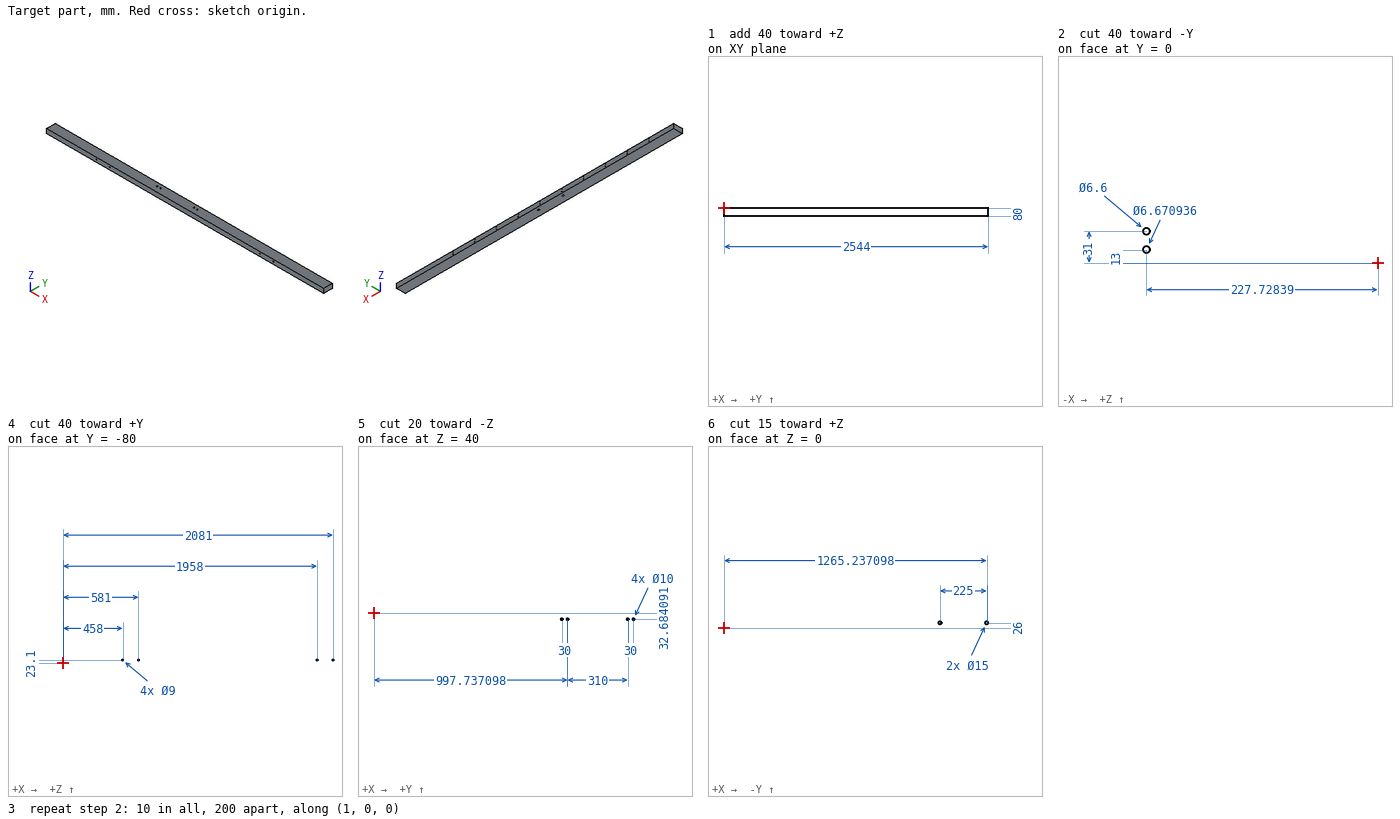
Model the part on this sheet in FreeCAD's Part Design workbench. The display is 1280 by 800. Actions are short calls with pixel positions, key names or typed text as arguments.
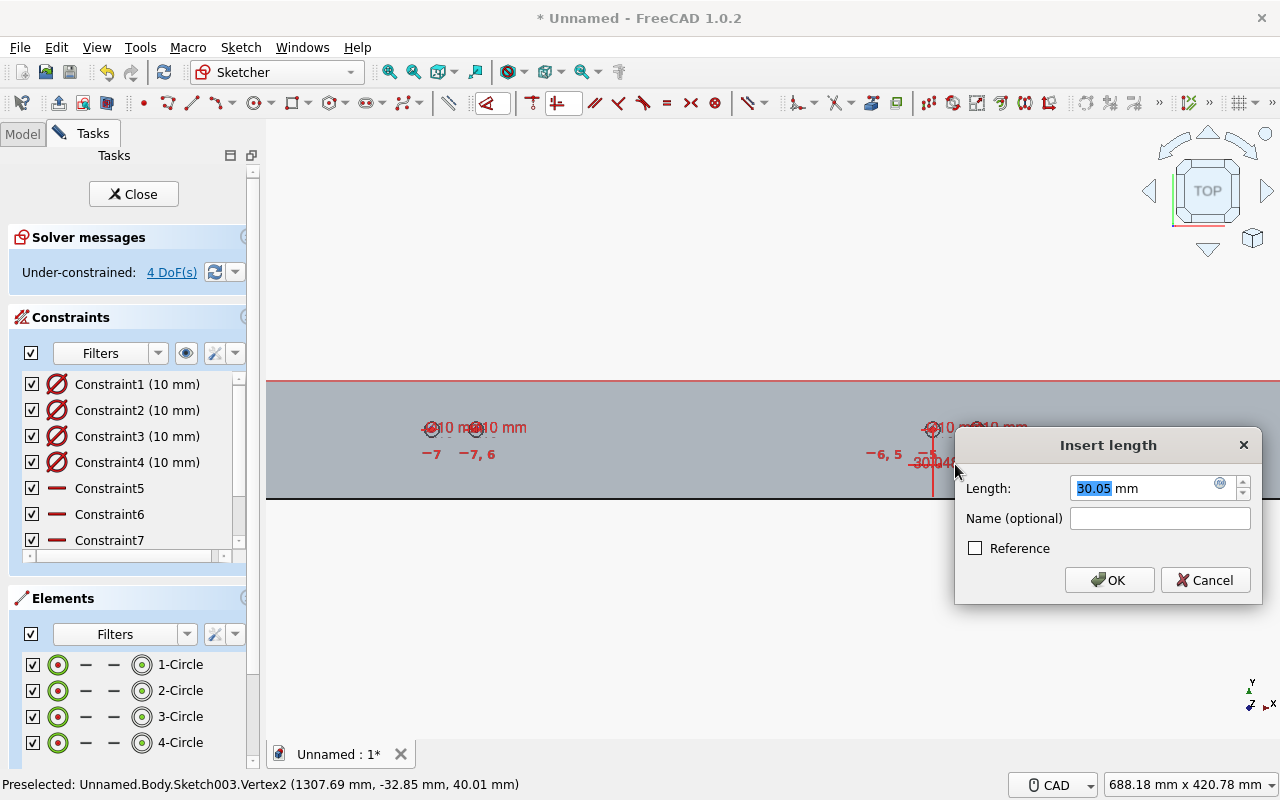
text(30)
key(Return)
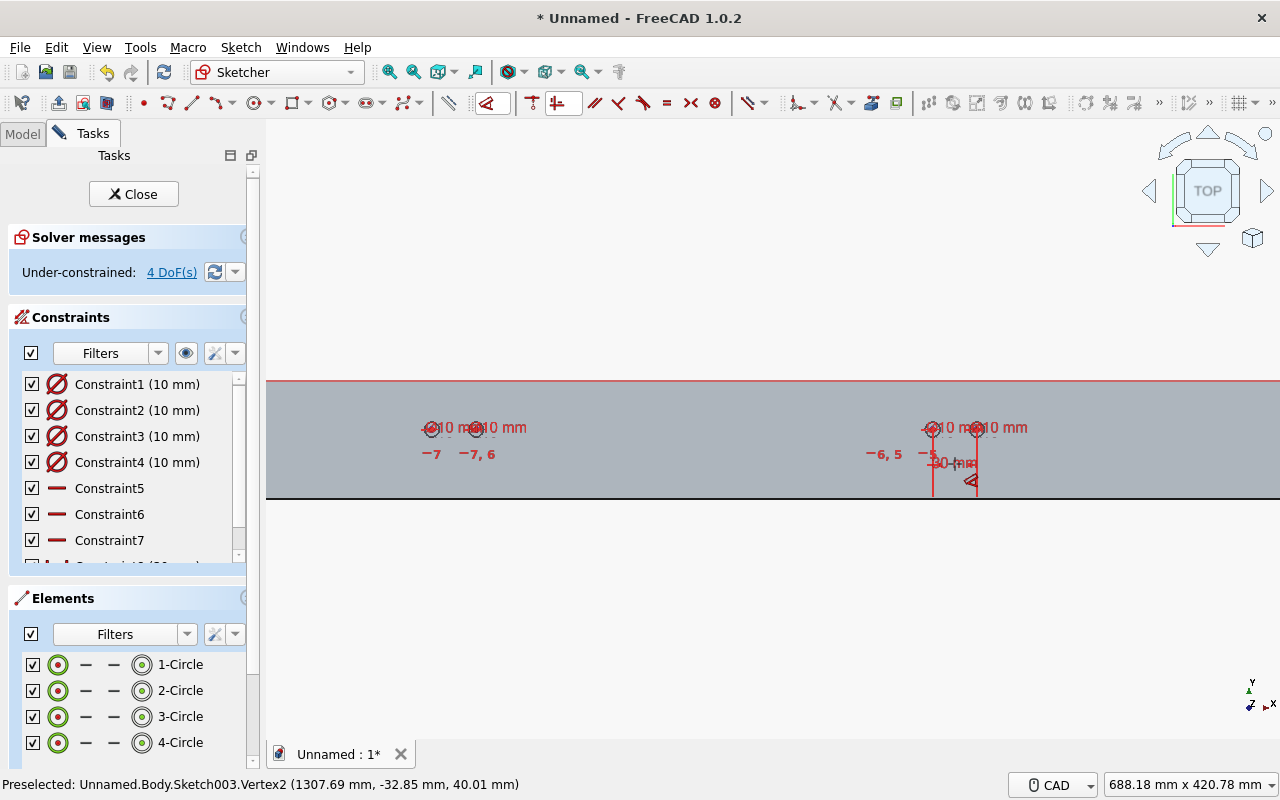
click(476, 430)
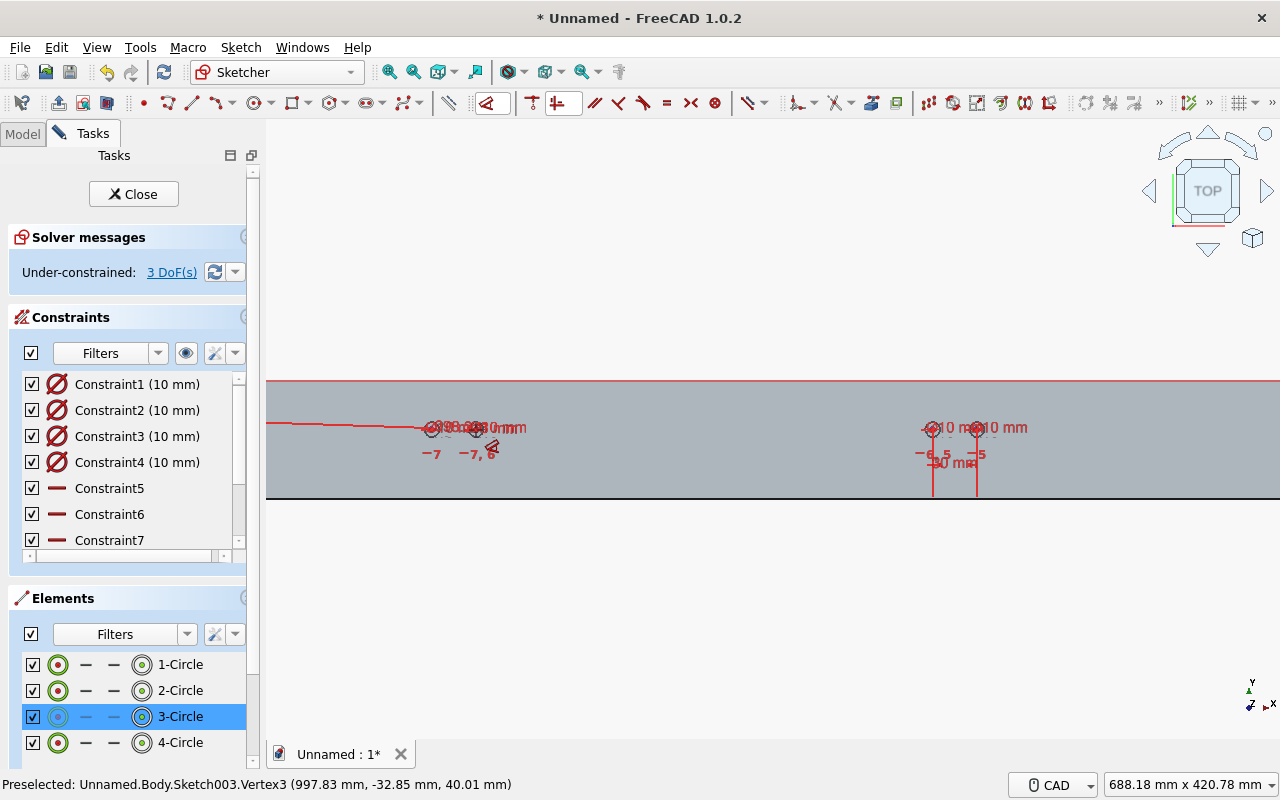
click(432, 430)
click(454, 464)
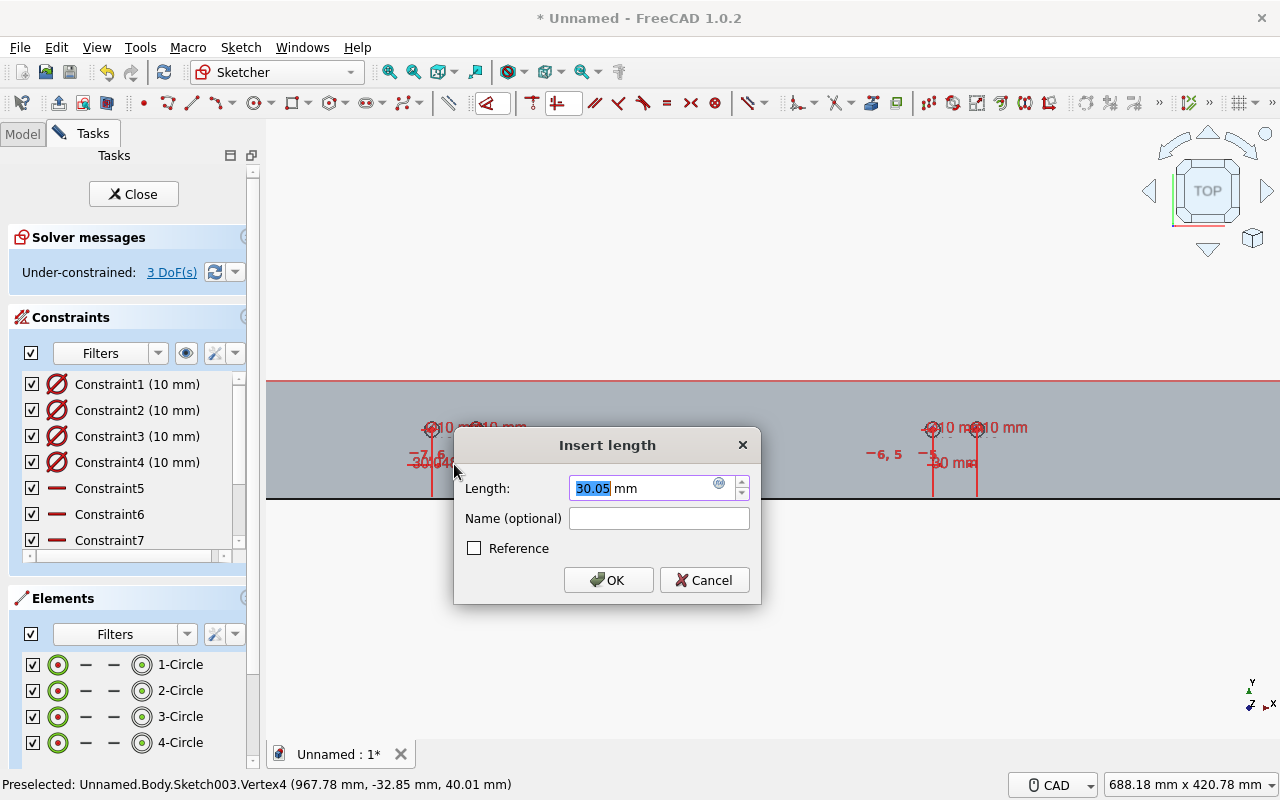
text(30)
key(Return)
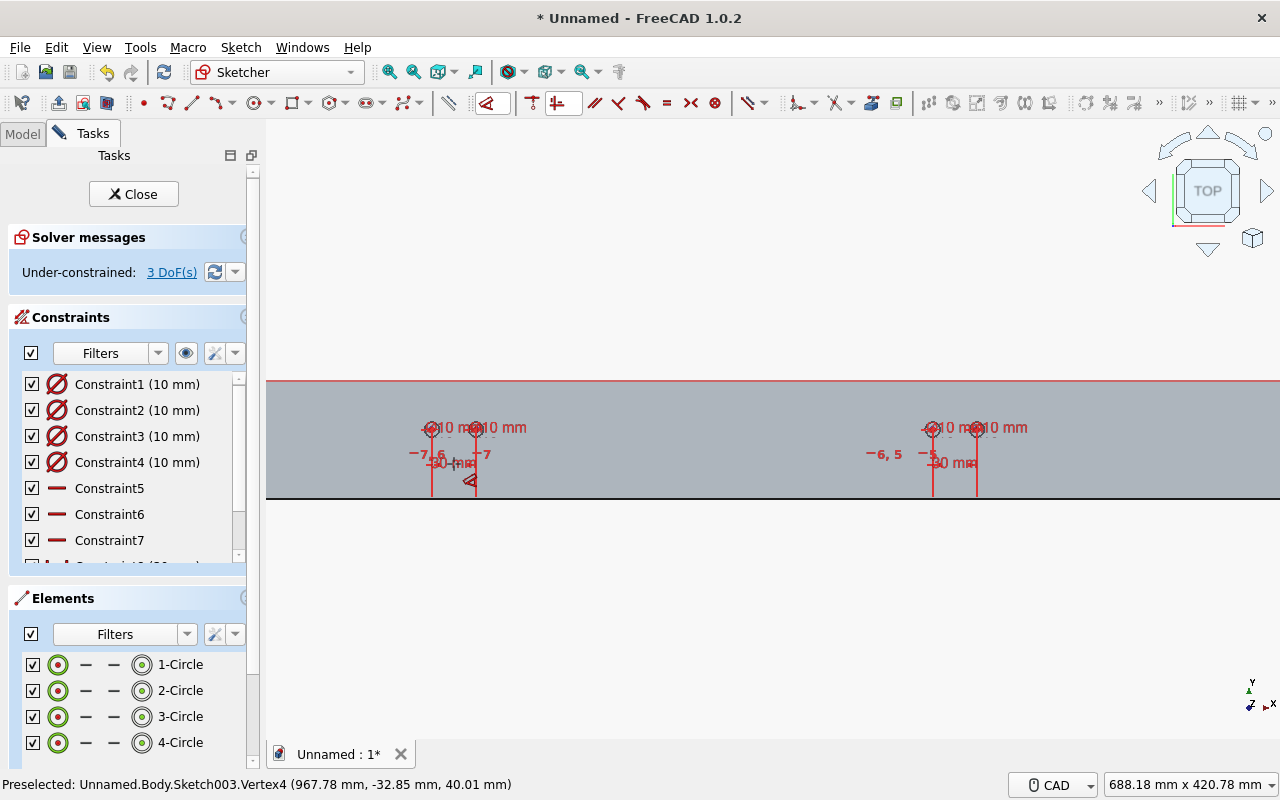
click(933, 430)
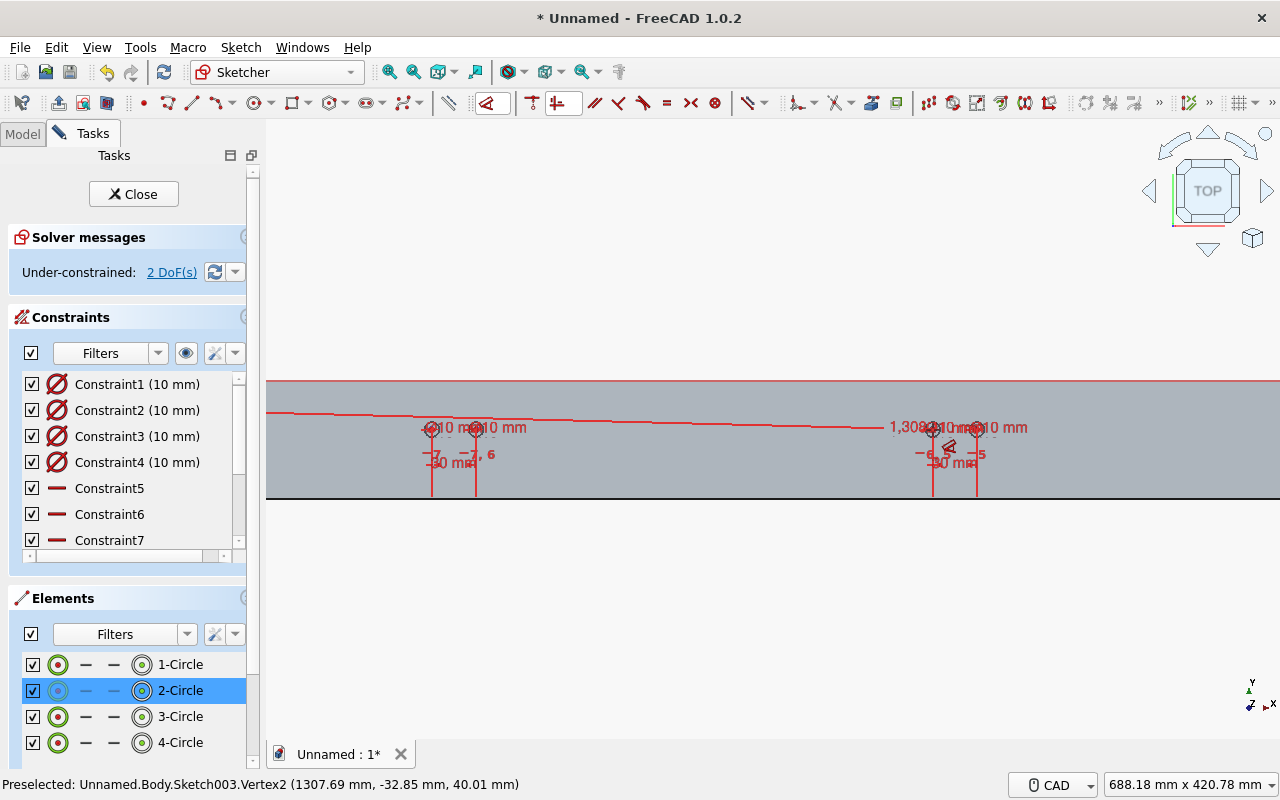
click(476, 430)
click(704, 464)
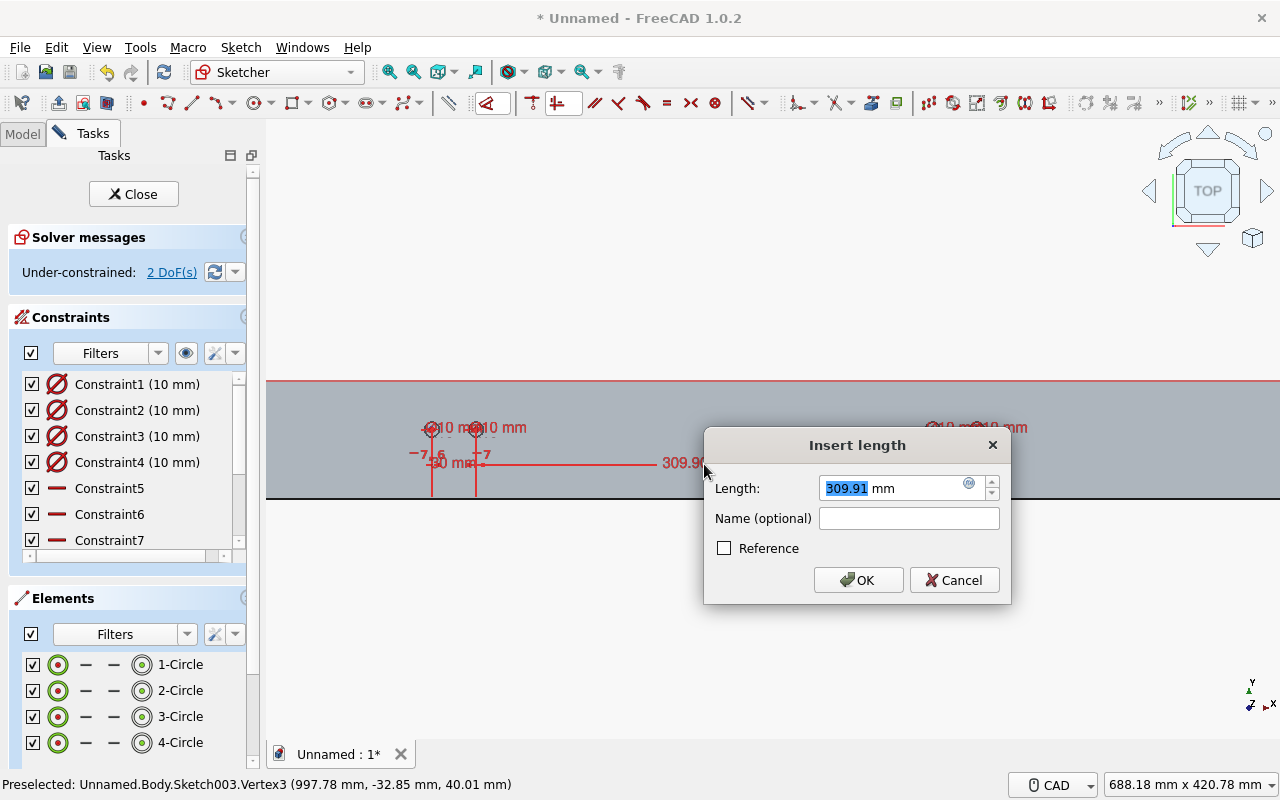
text(310)
key(Return)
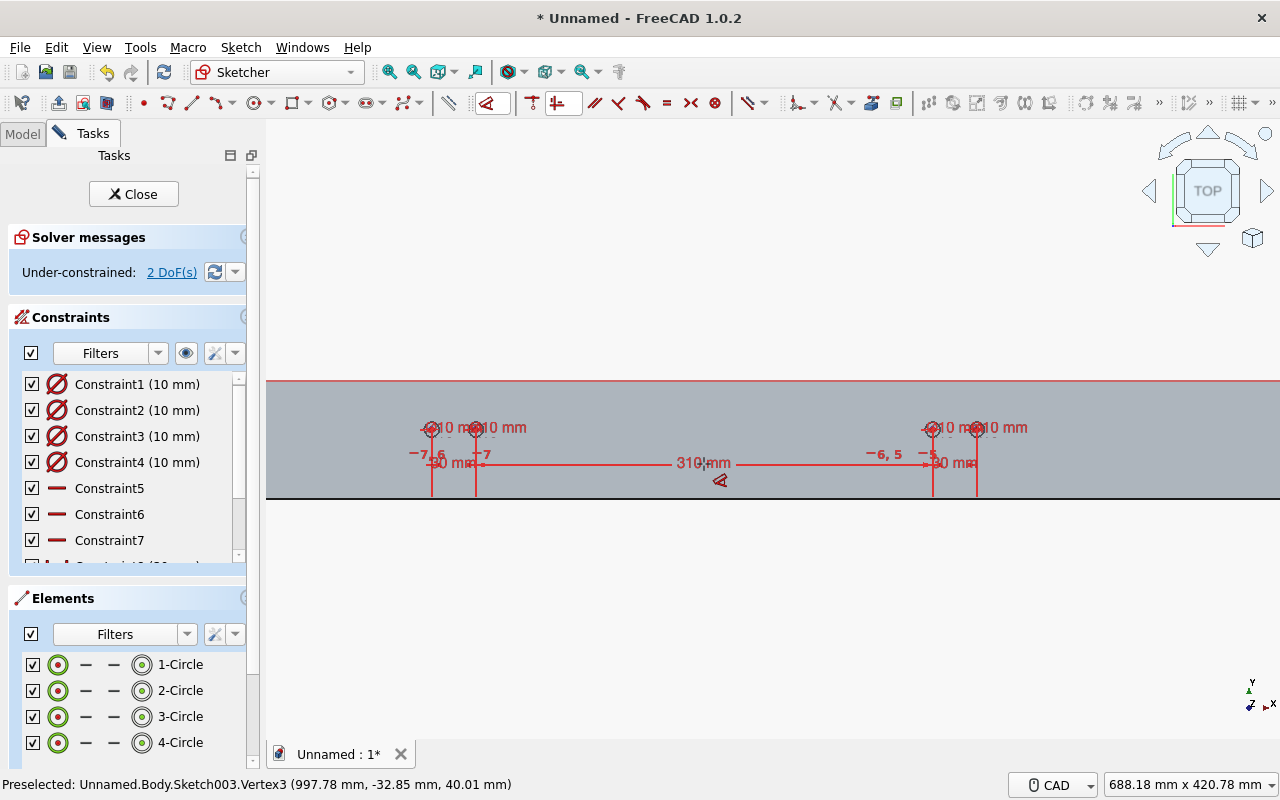
click(977, 430)
click(1011, 405)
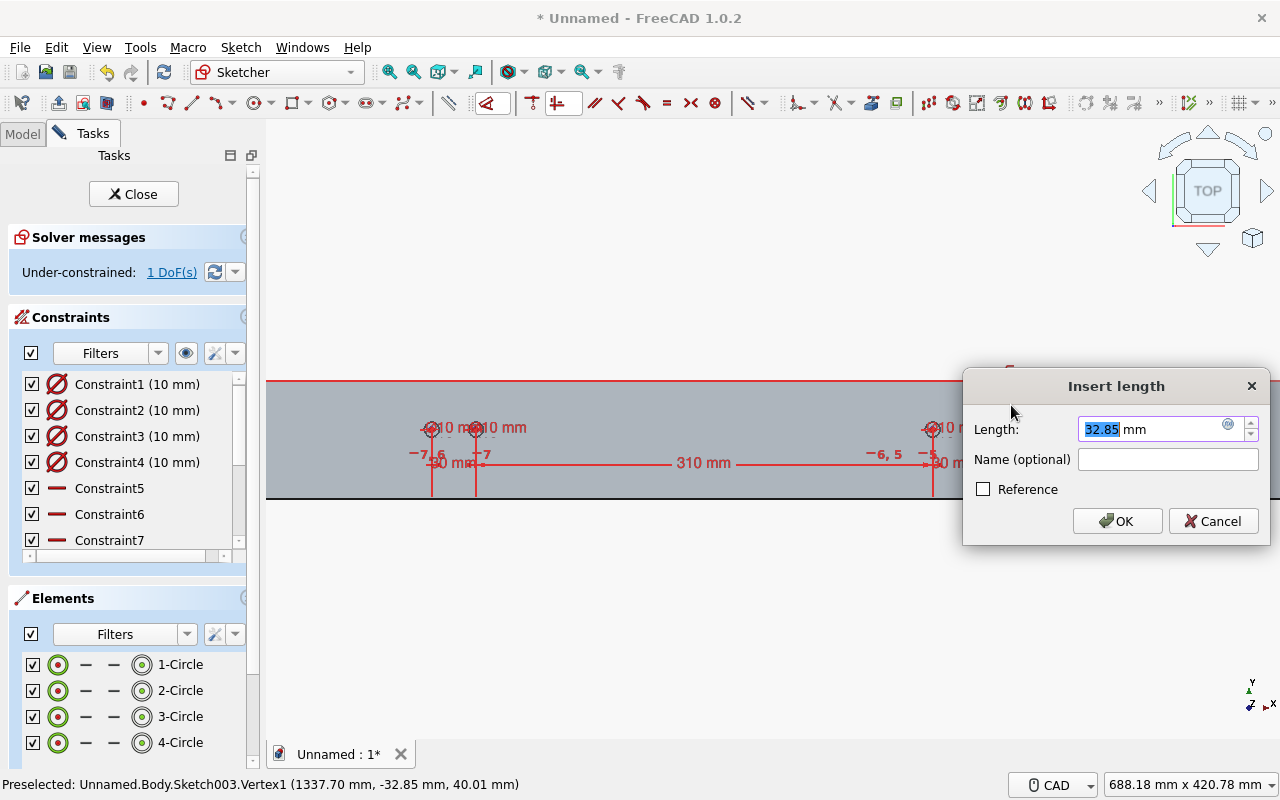
text(32.684091)
key(Return)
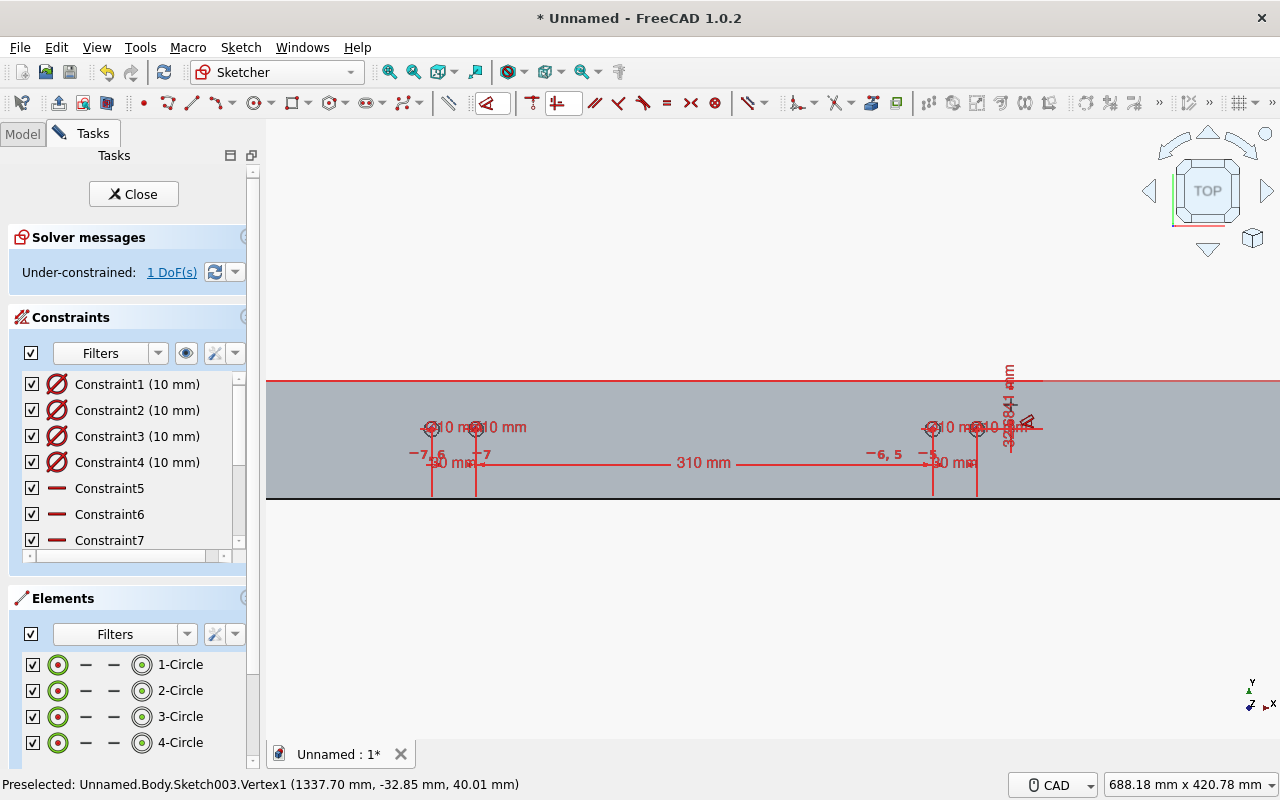
click(476, 429)
click(385, 347)